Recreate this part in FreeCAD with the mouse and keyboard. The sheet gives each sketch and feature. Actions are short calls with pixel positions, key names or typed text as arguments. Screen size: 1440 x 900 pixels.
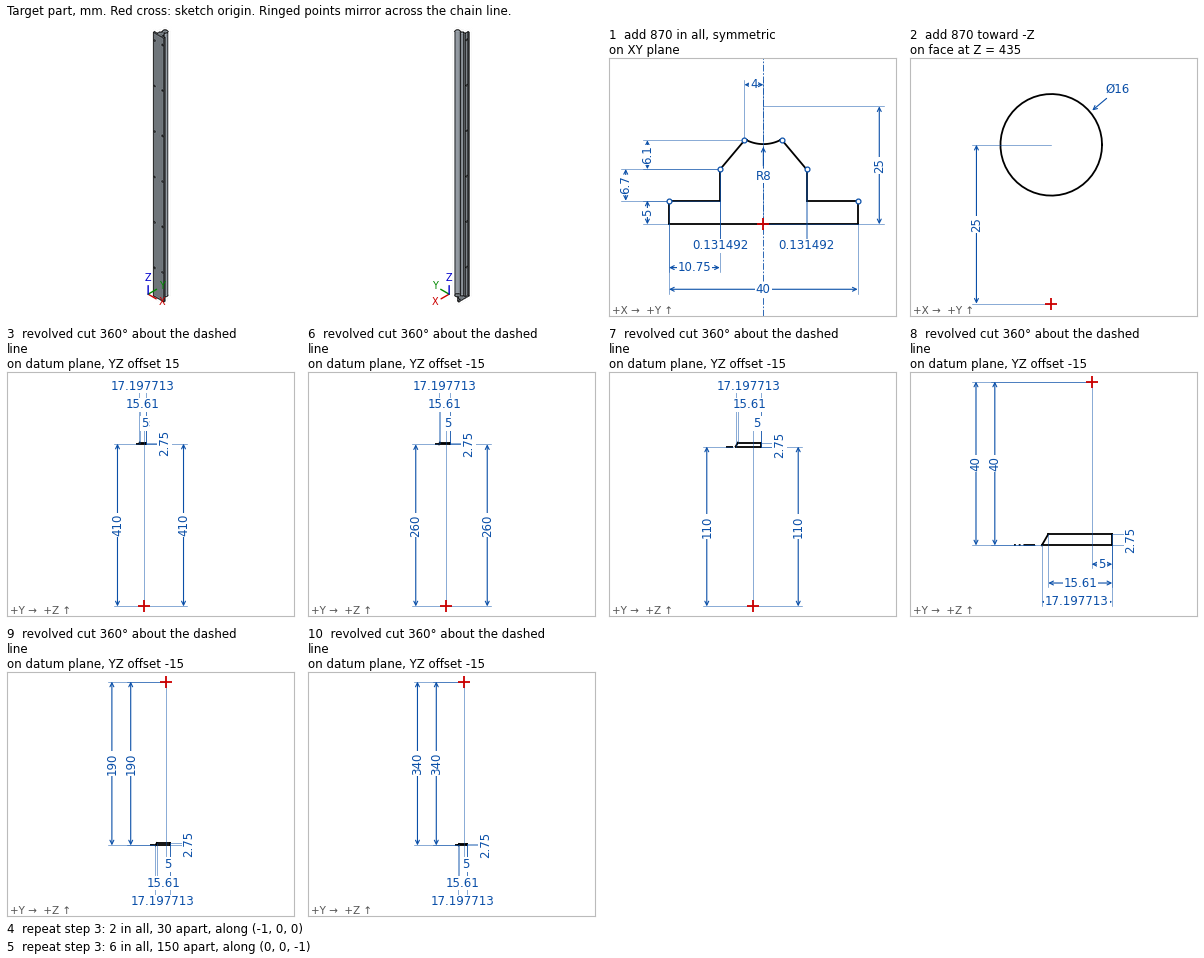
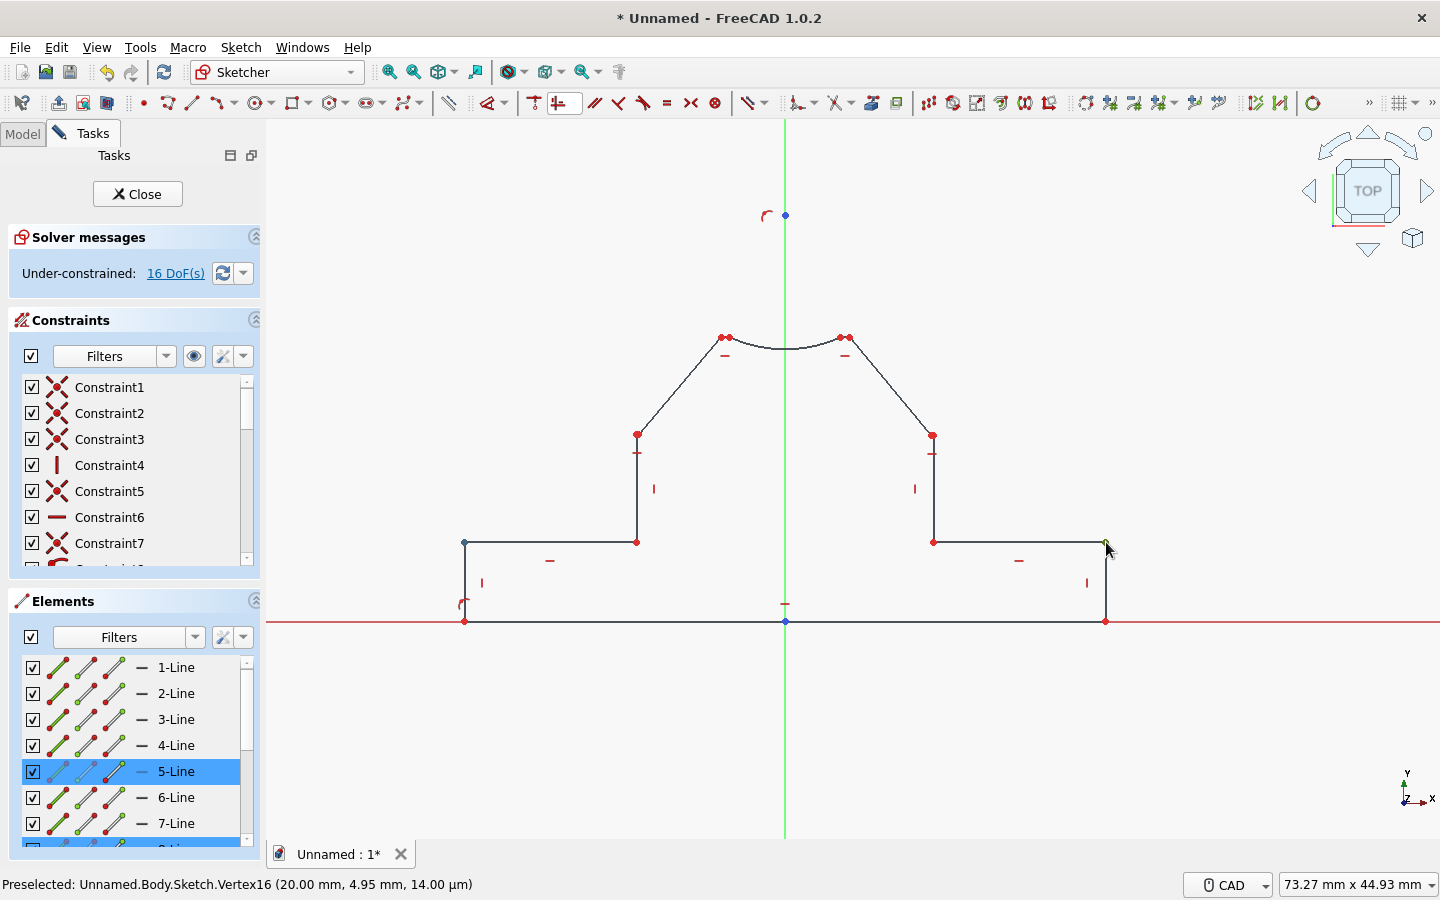
click(785, 764)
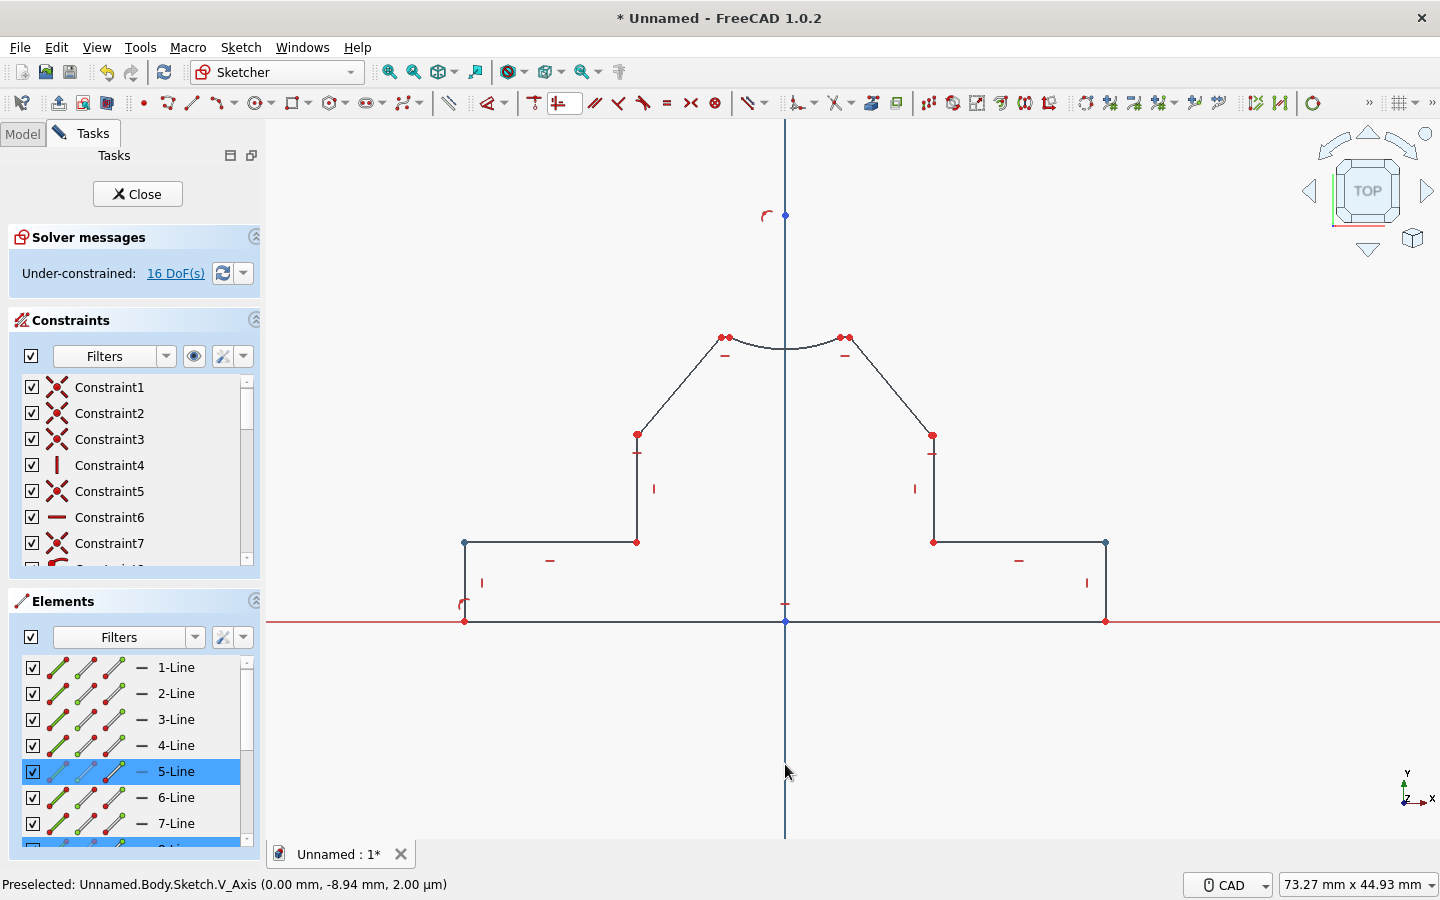
click(692, 104)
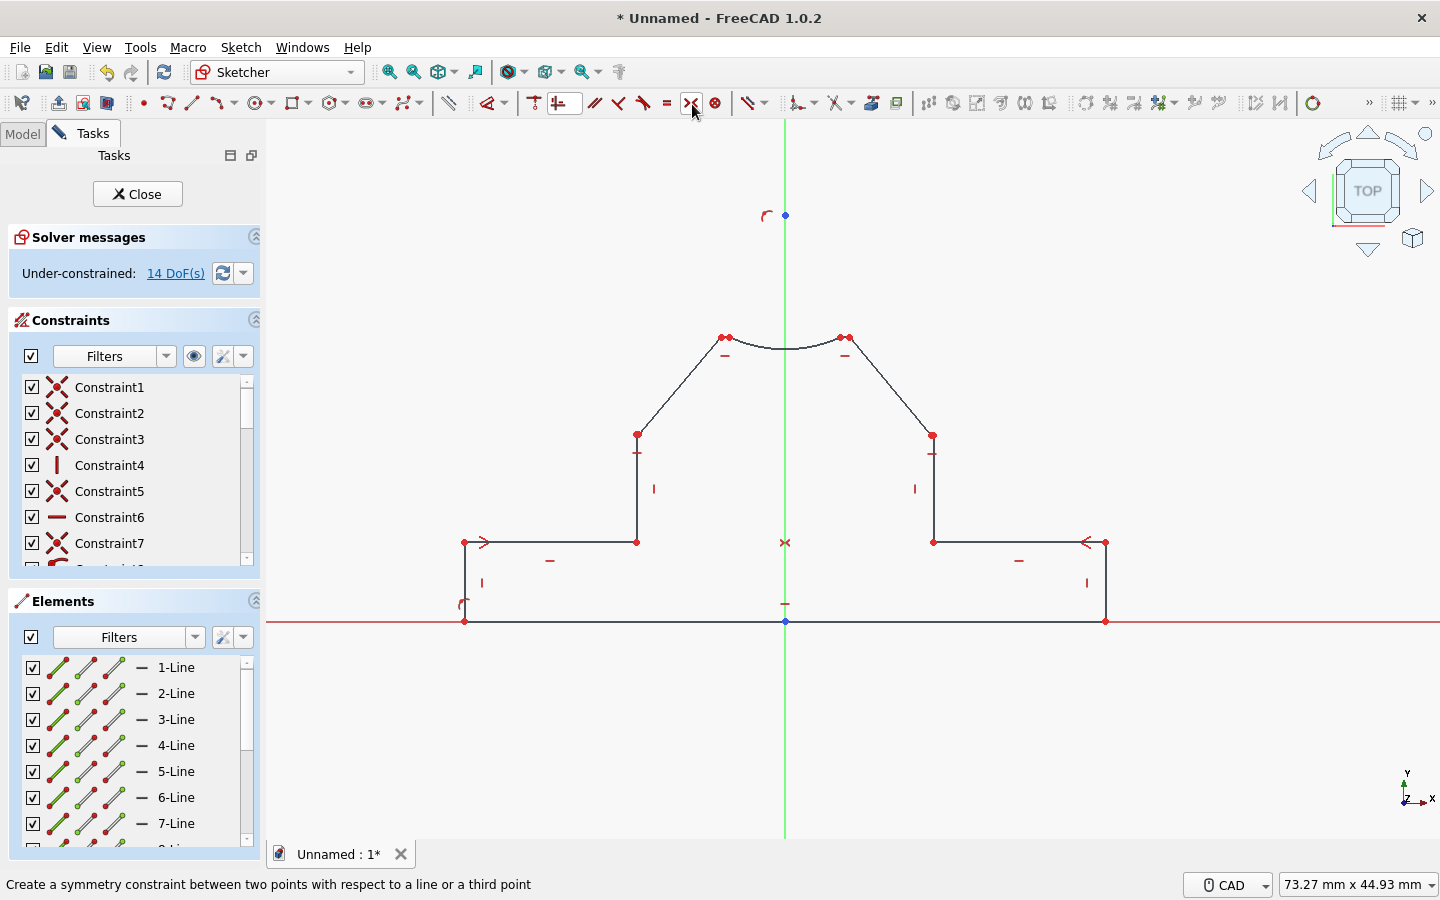
scroll(637, 435, up, 9)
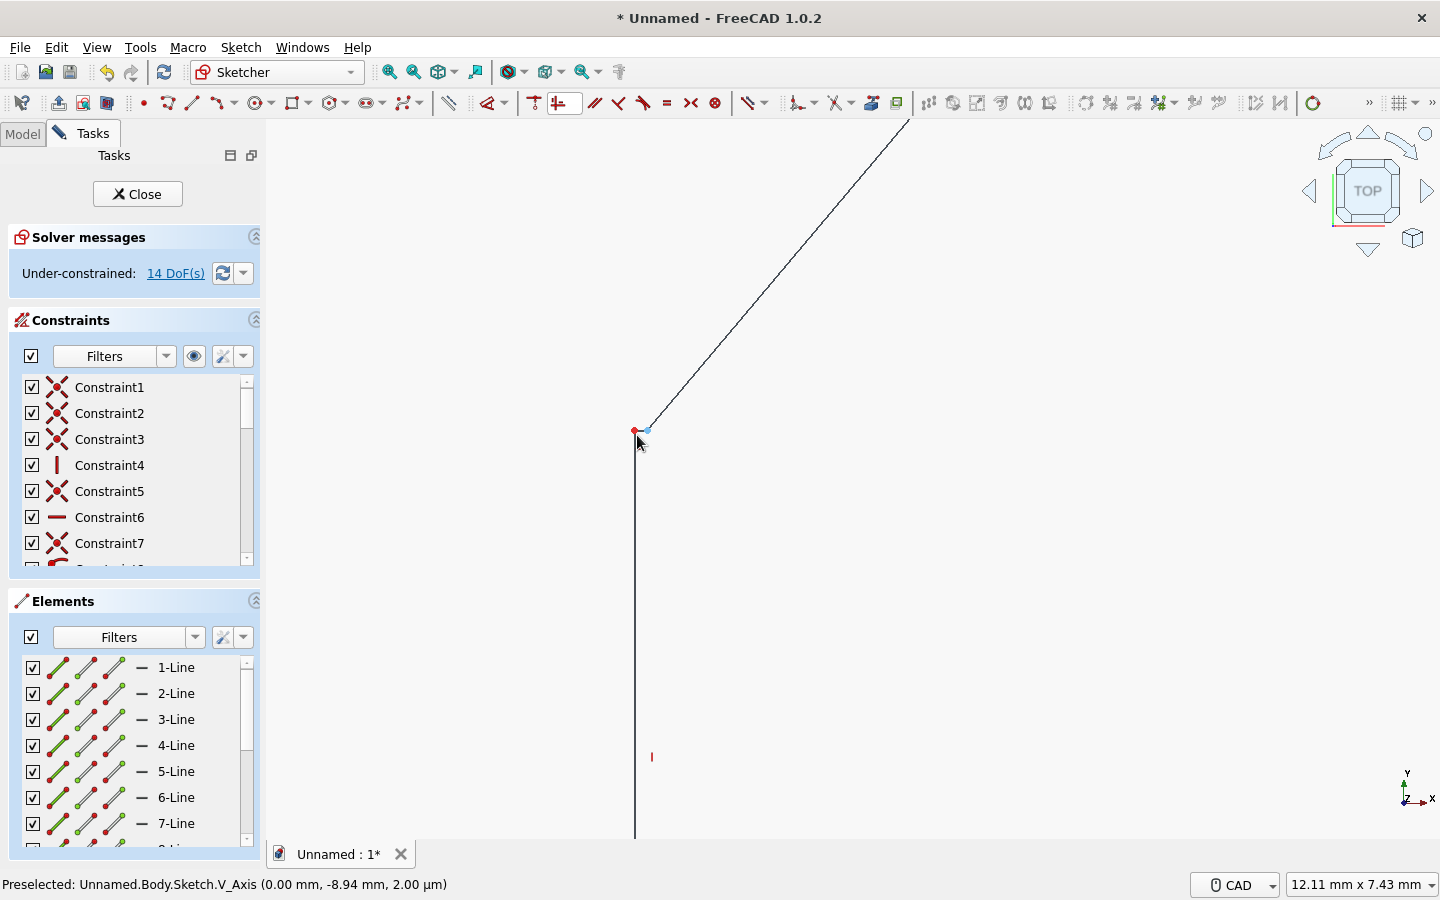
click(635, 431)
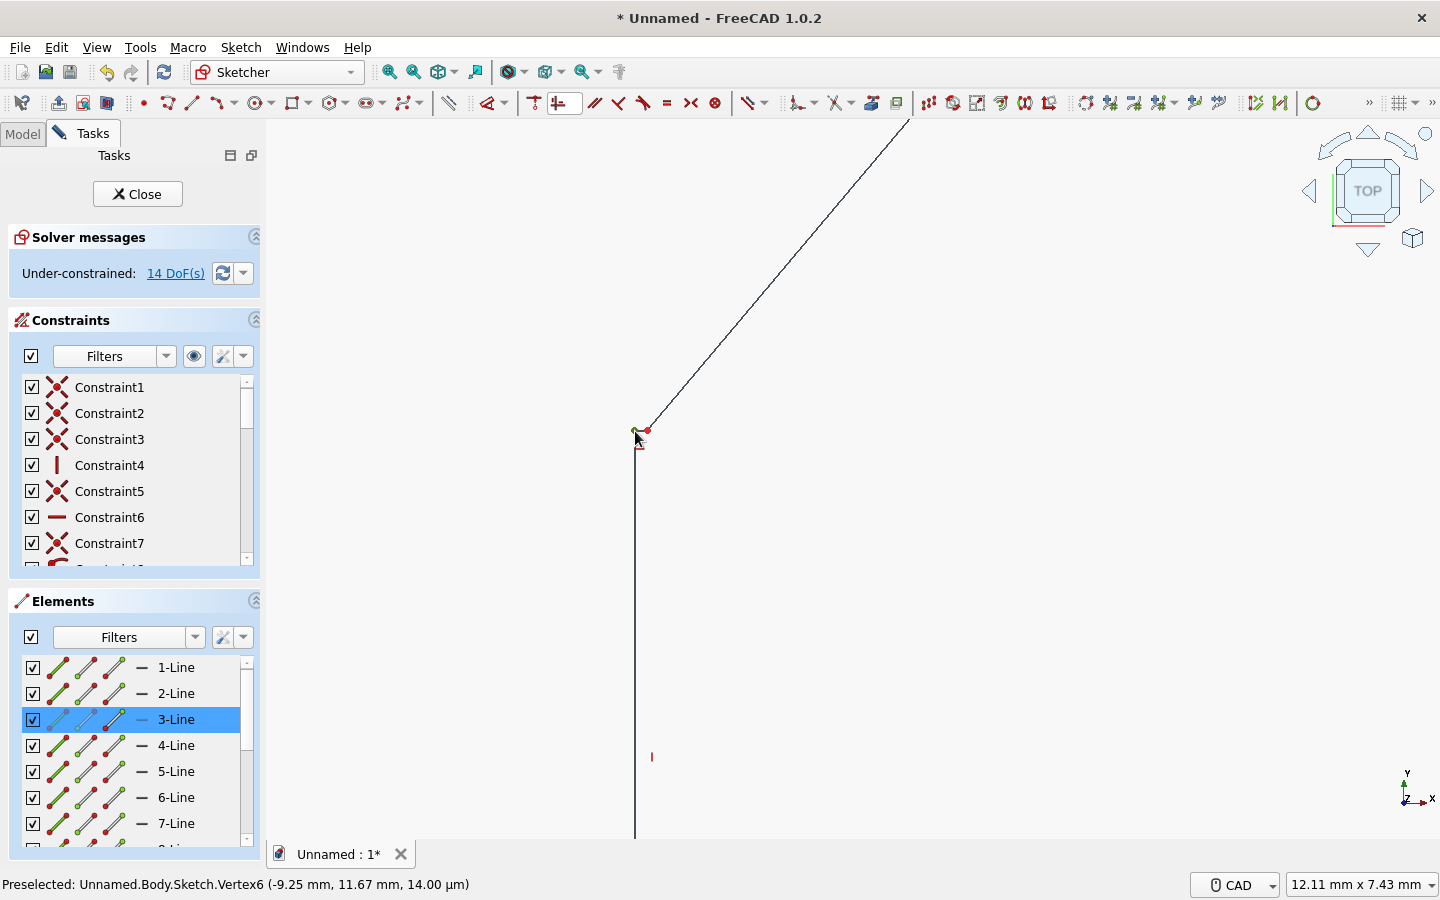
scroll(637, 435, down, 9)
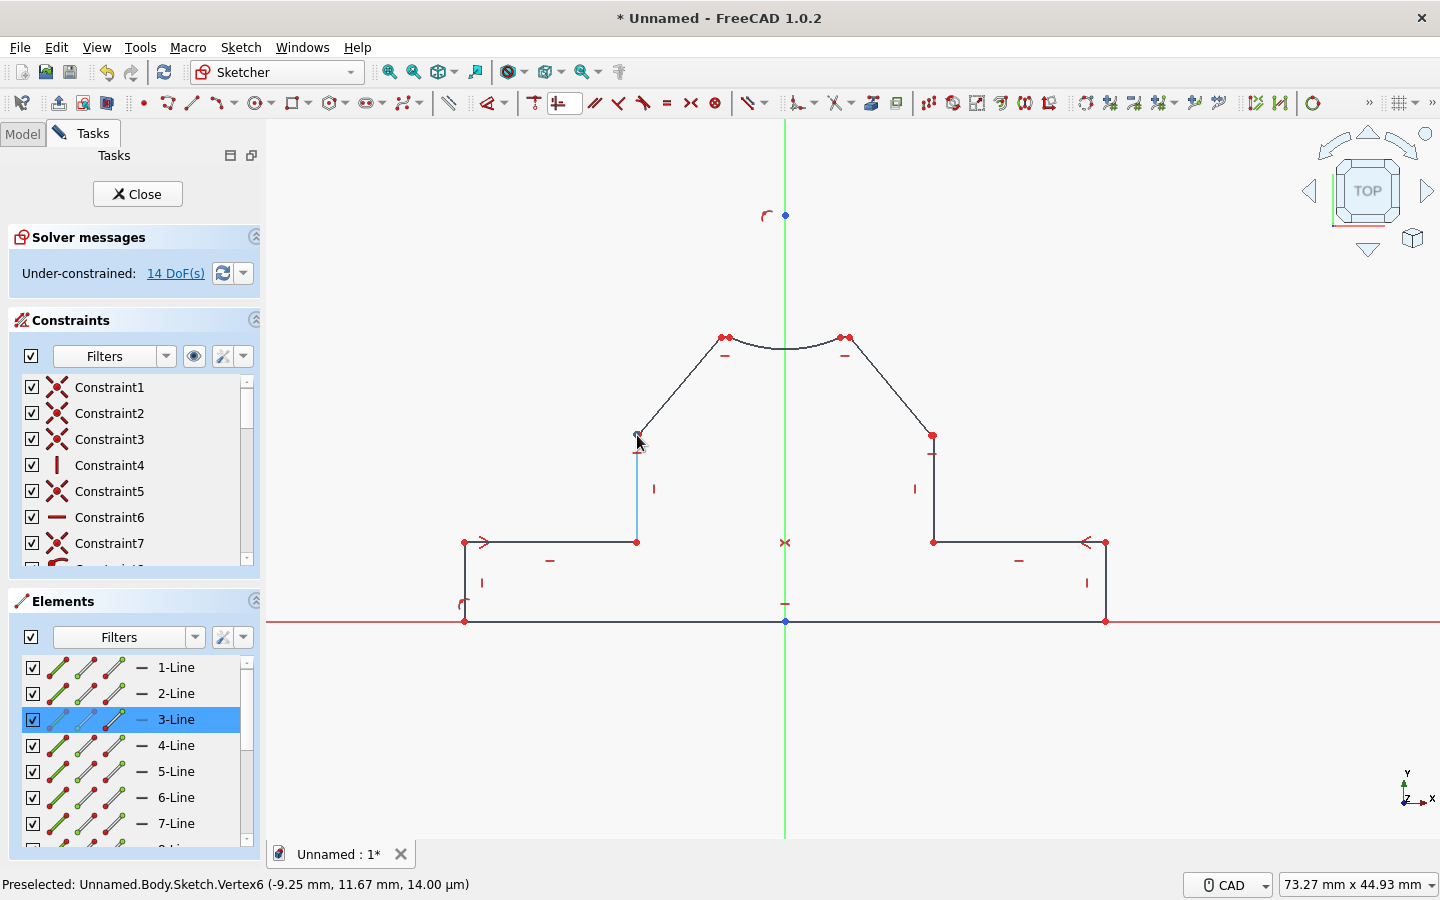
scroll(934, 435, up, 9)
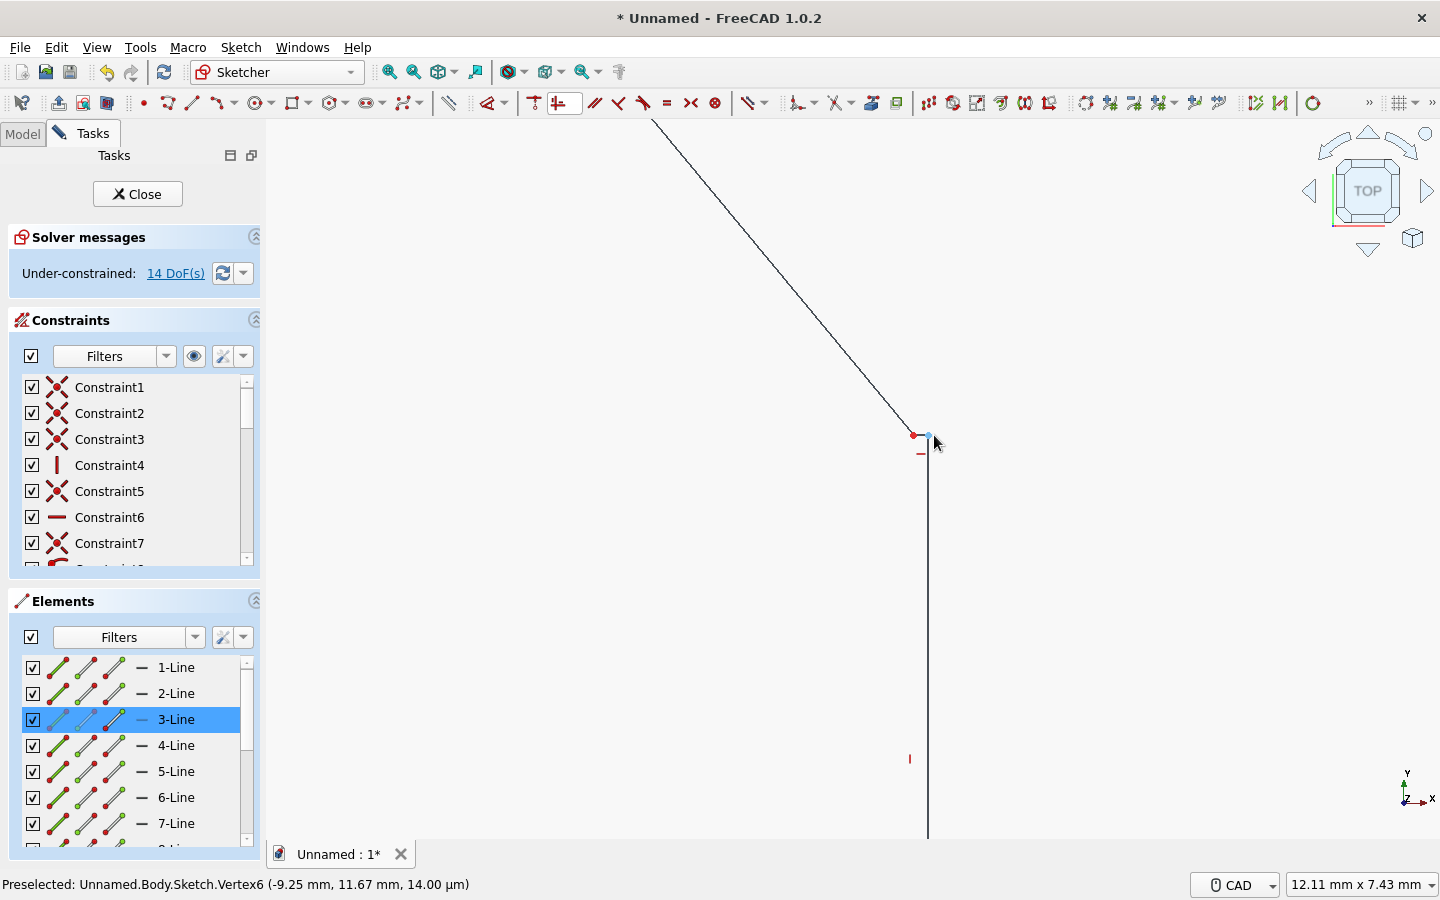
click(928, 435)